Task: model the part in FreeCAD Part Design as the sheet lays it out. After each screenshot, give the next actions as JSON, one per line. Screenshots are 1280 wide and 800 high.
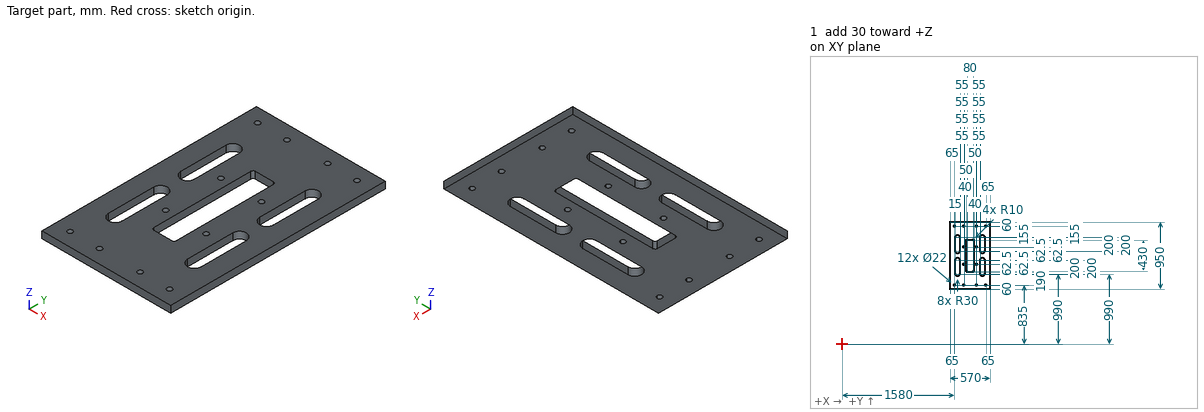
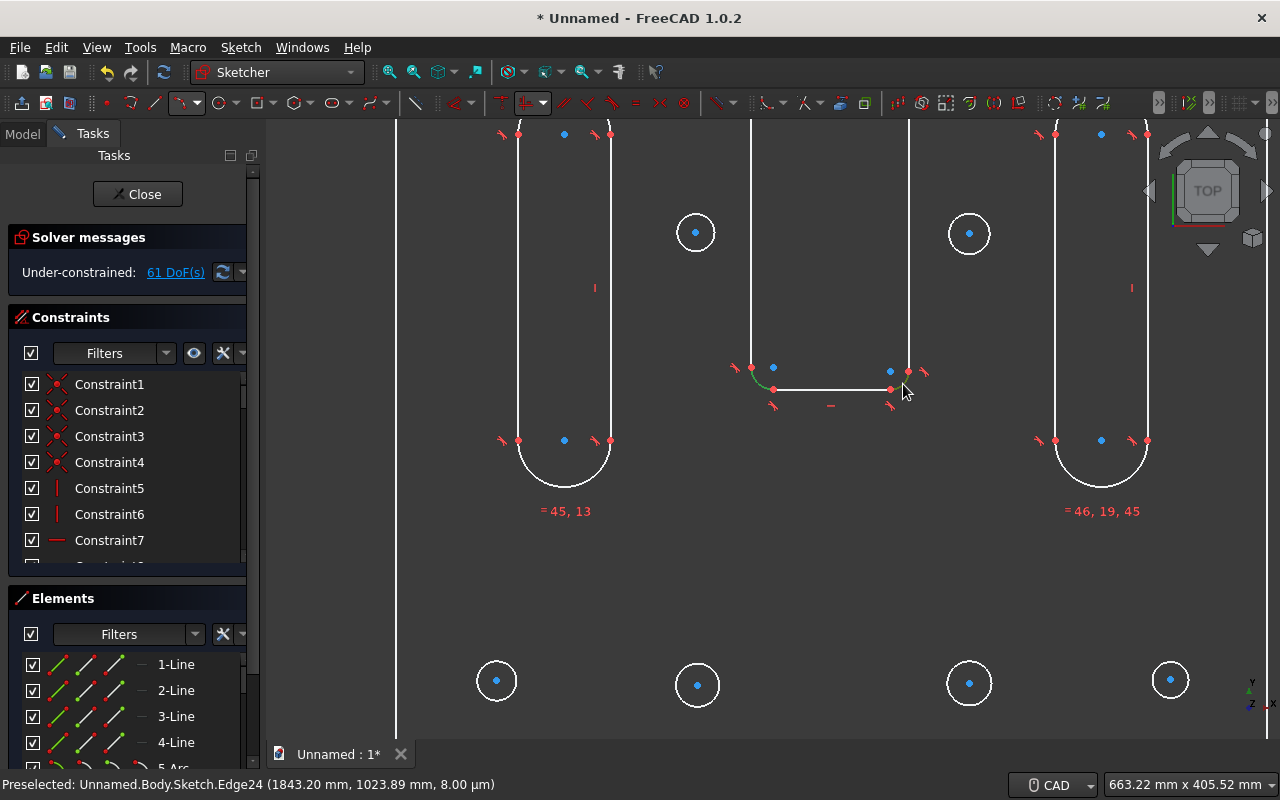
{"action": "left_click", "coordinate": [636, 104]}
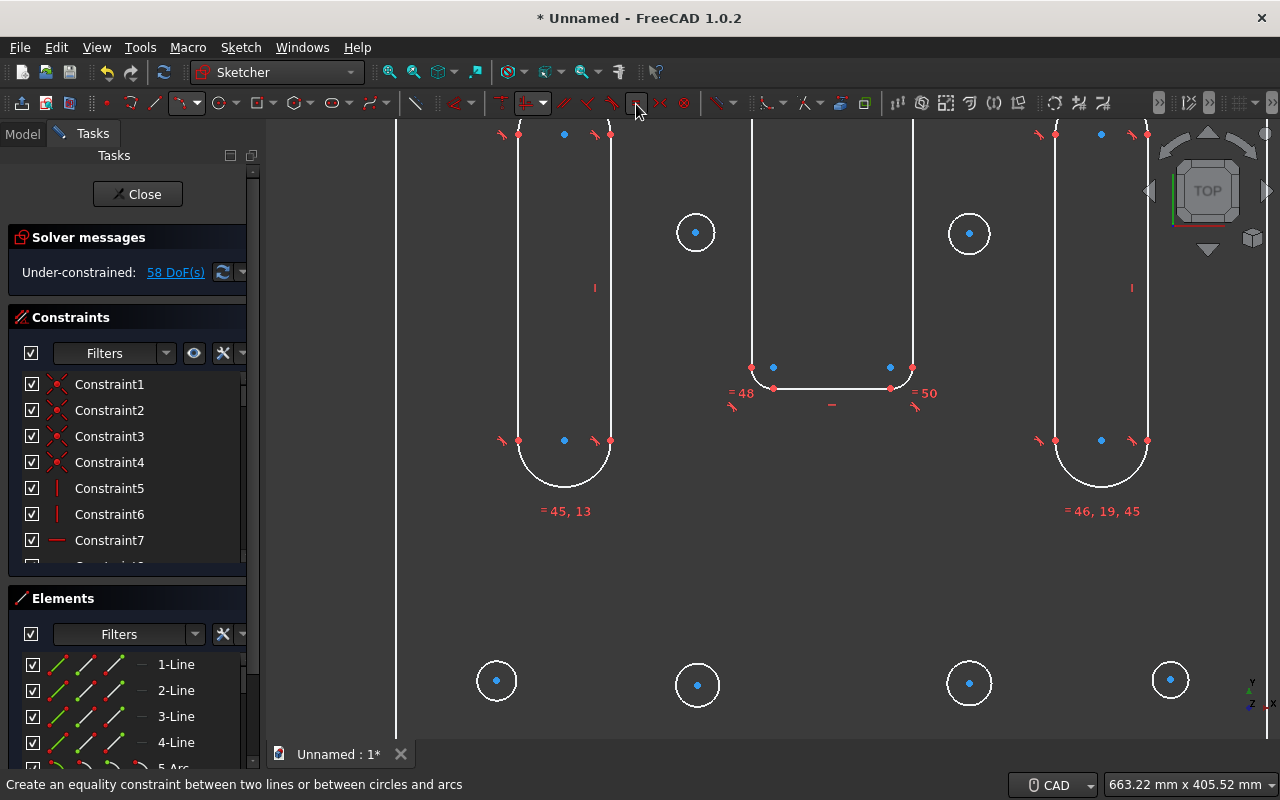
{"action": "left_click", "coordinate": [511, 667]}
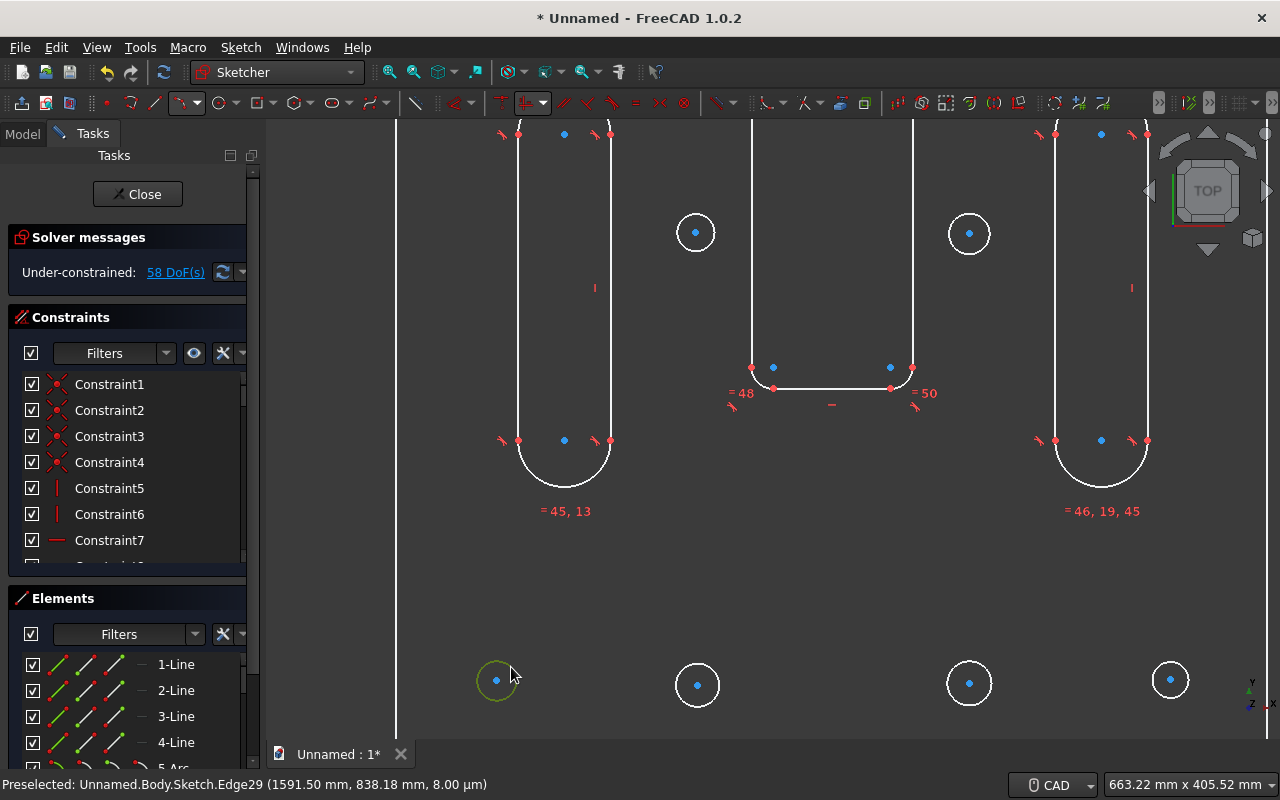
{"action": "left_click", "coordinate": [713, 670]}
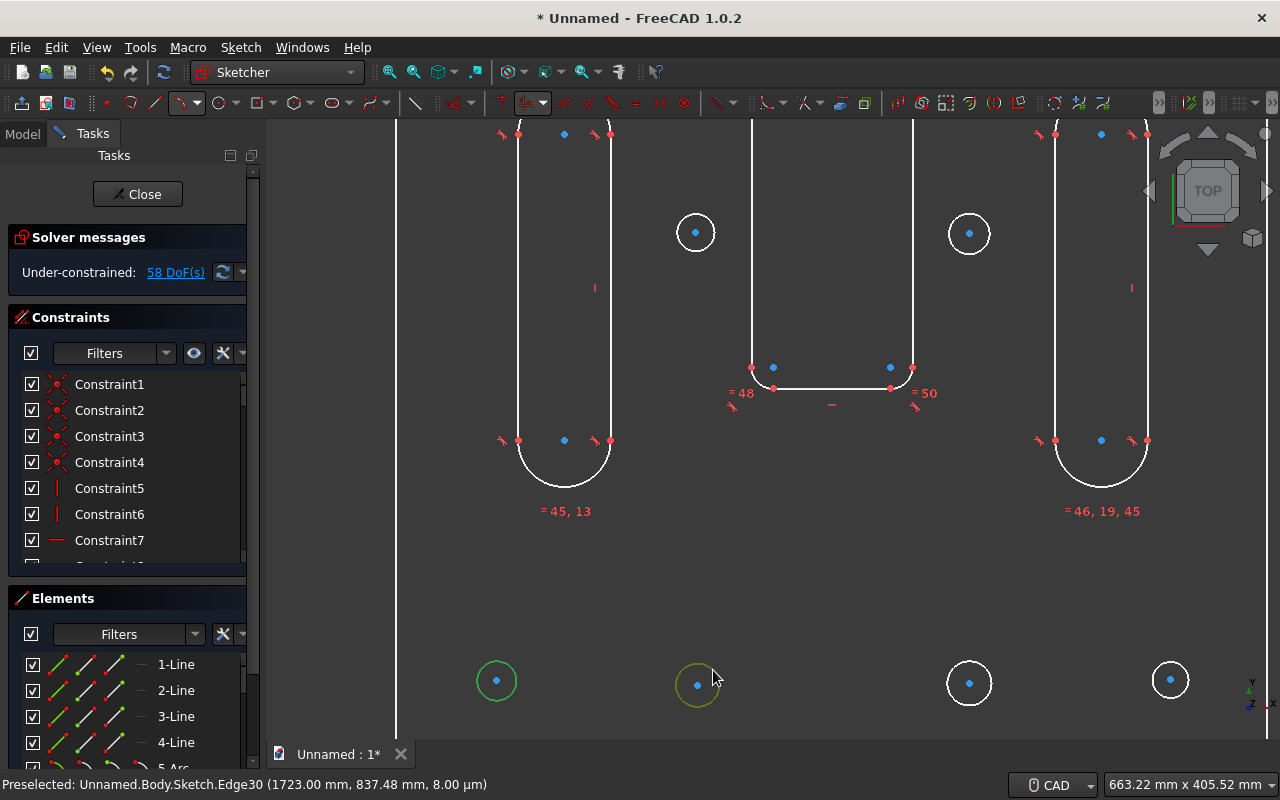
{"action": "left_click", "coordinate": [709, 219]}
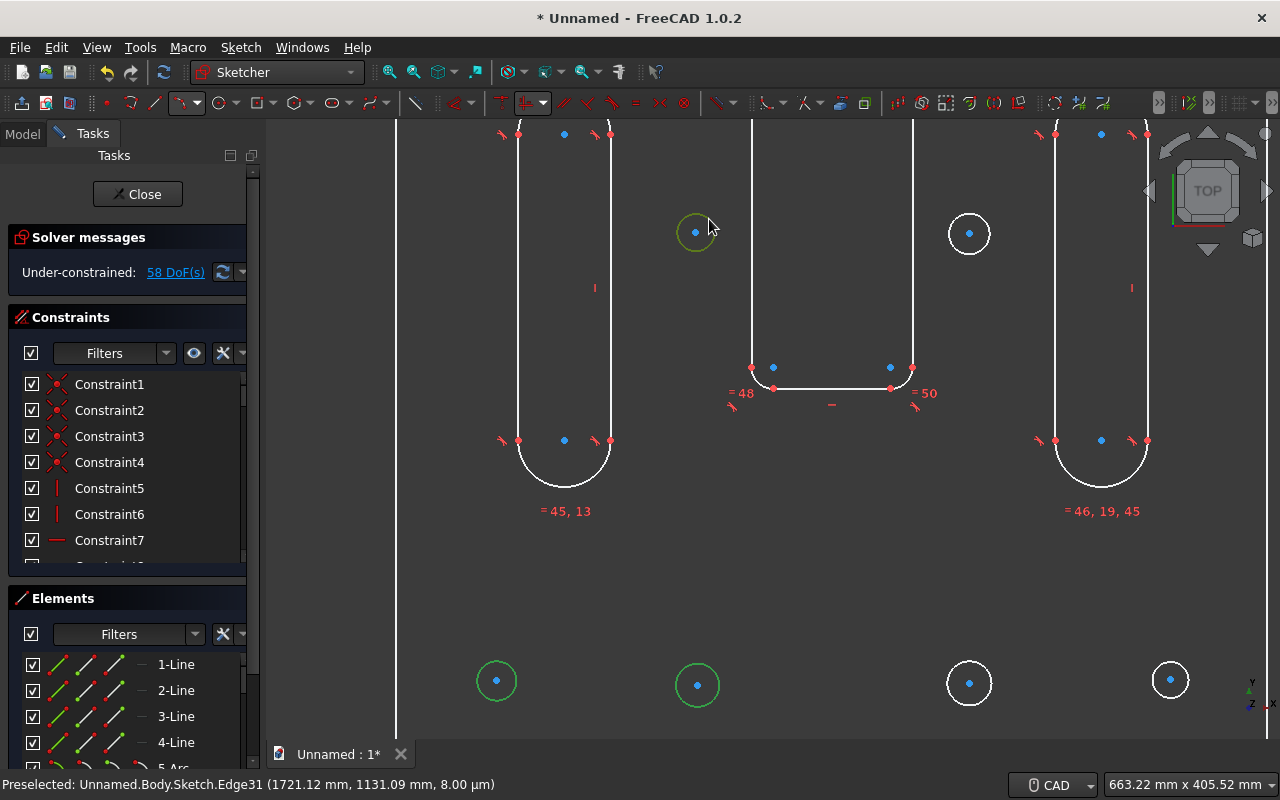
{"action": "left_click", "coordinate": [985, 668]}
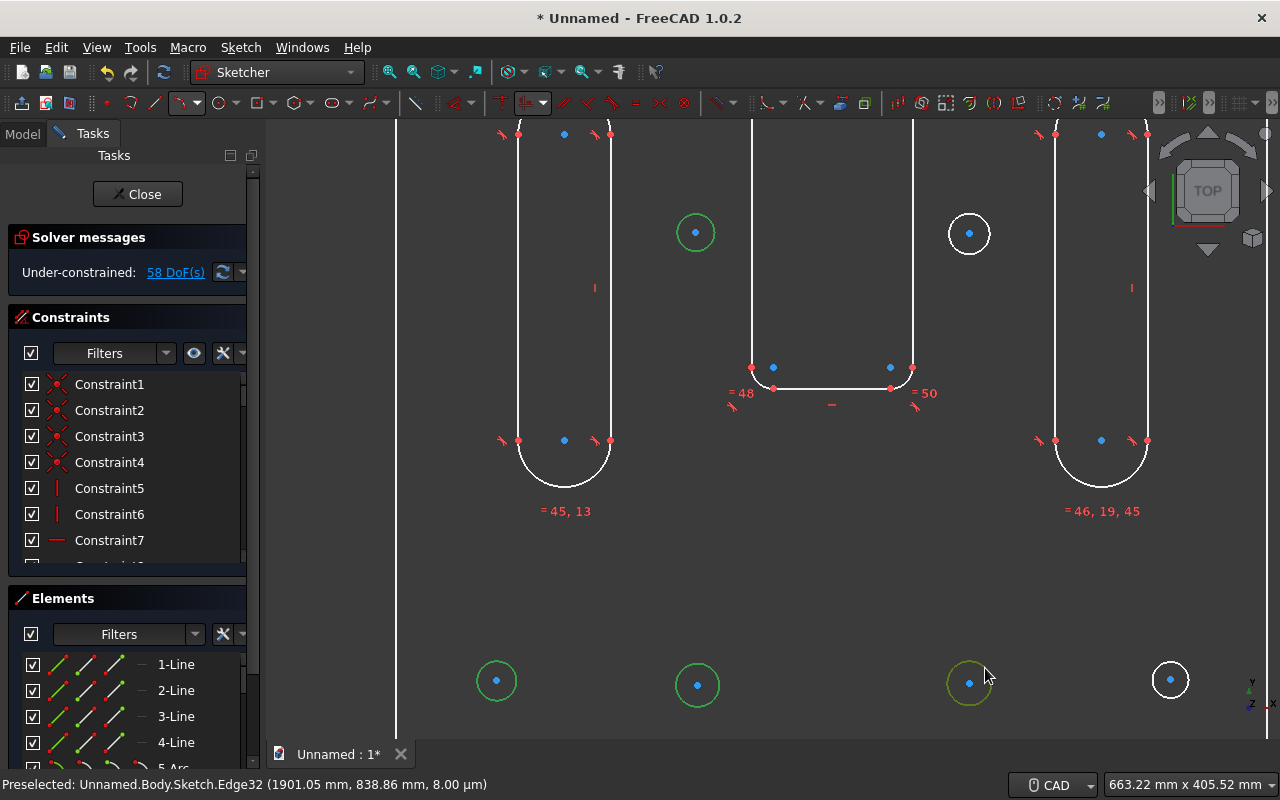
{"action": "scroll", "coordinate": [908, 388], "scroll_direction": "down", "scroll_amount": 9}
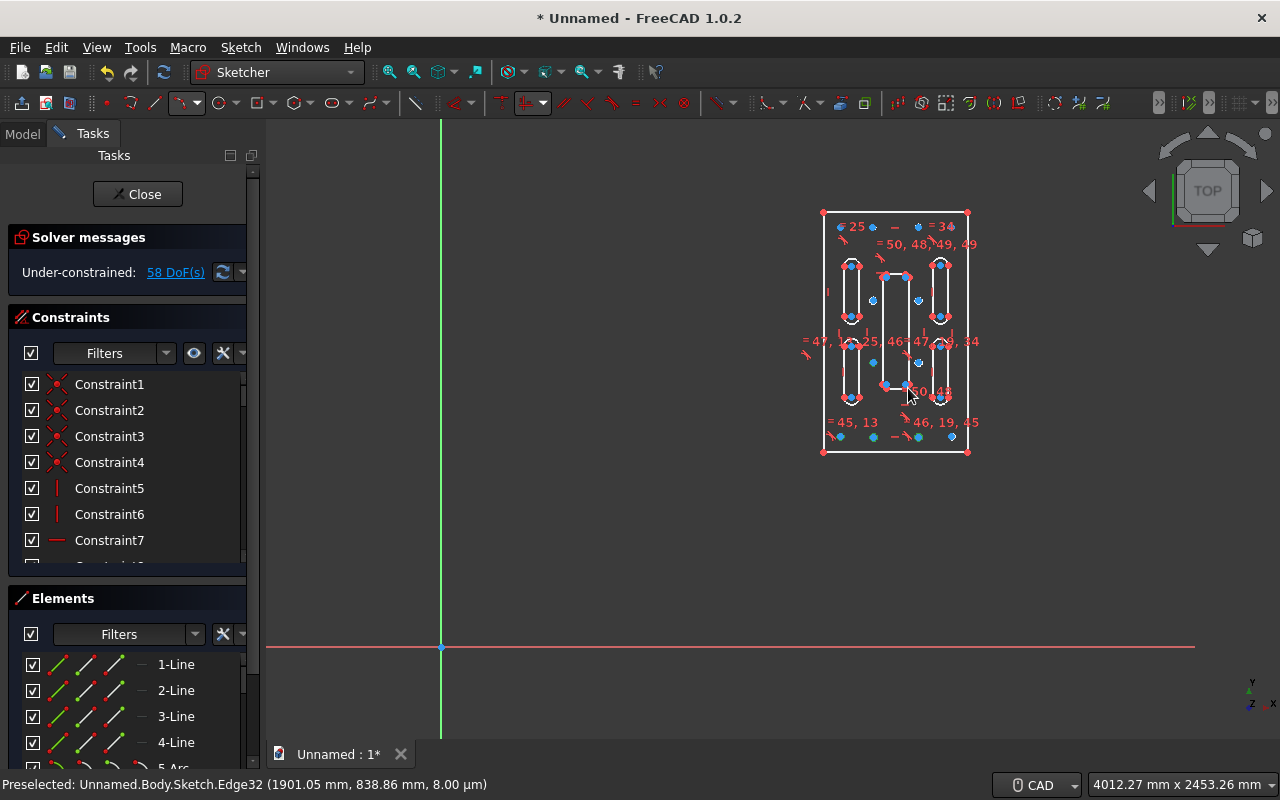
{"action": "scroll", "coordinate": [954, 435], "scroll_direction": "up", "scroll_amount": 8}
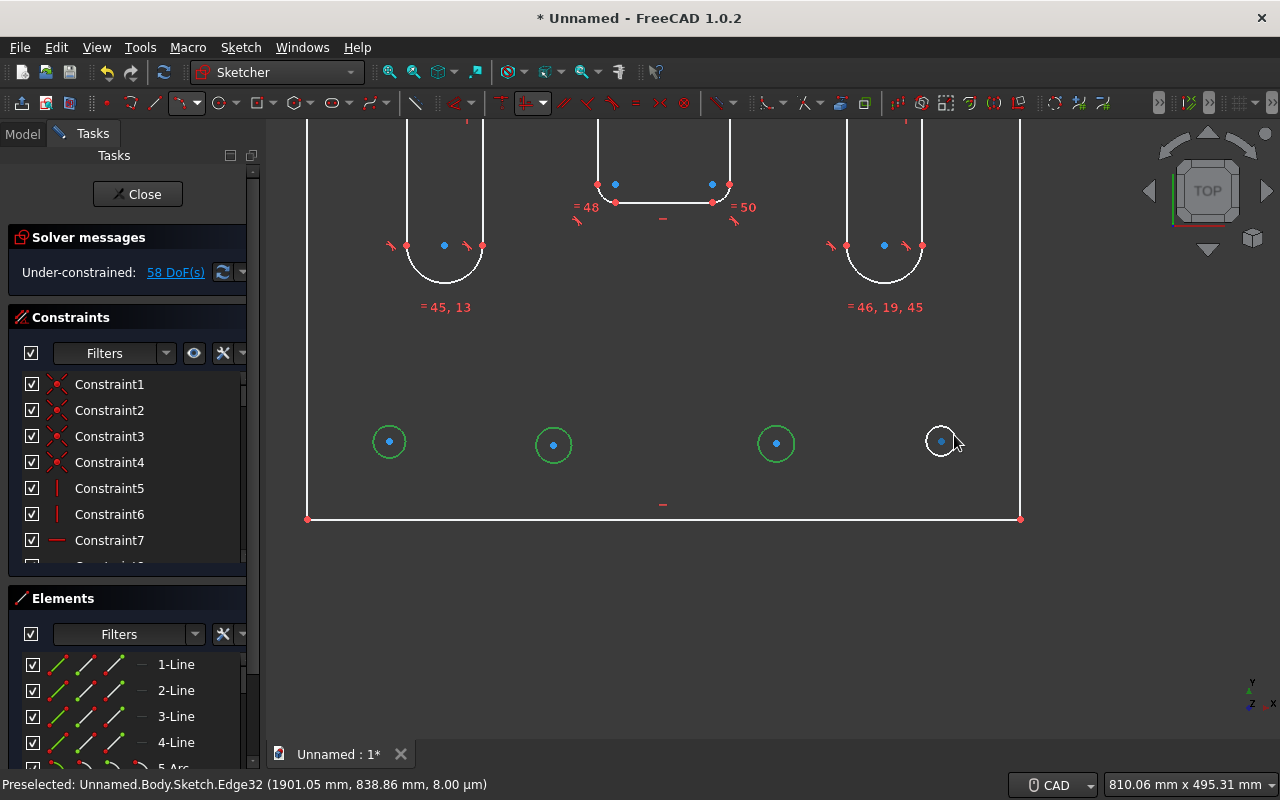
{"action": "left_click", "coordinate": [951, 431]}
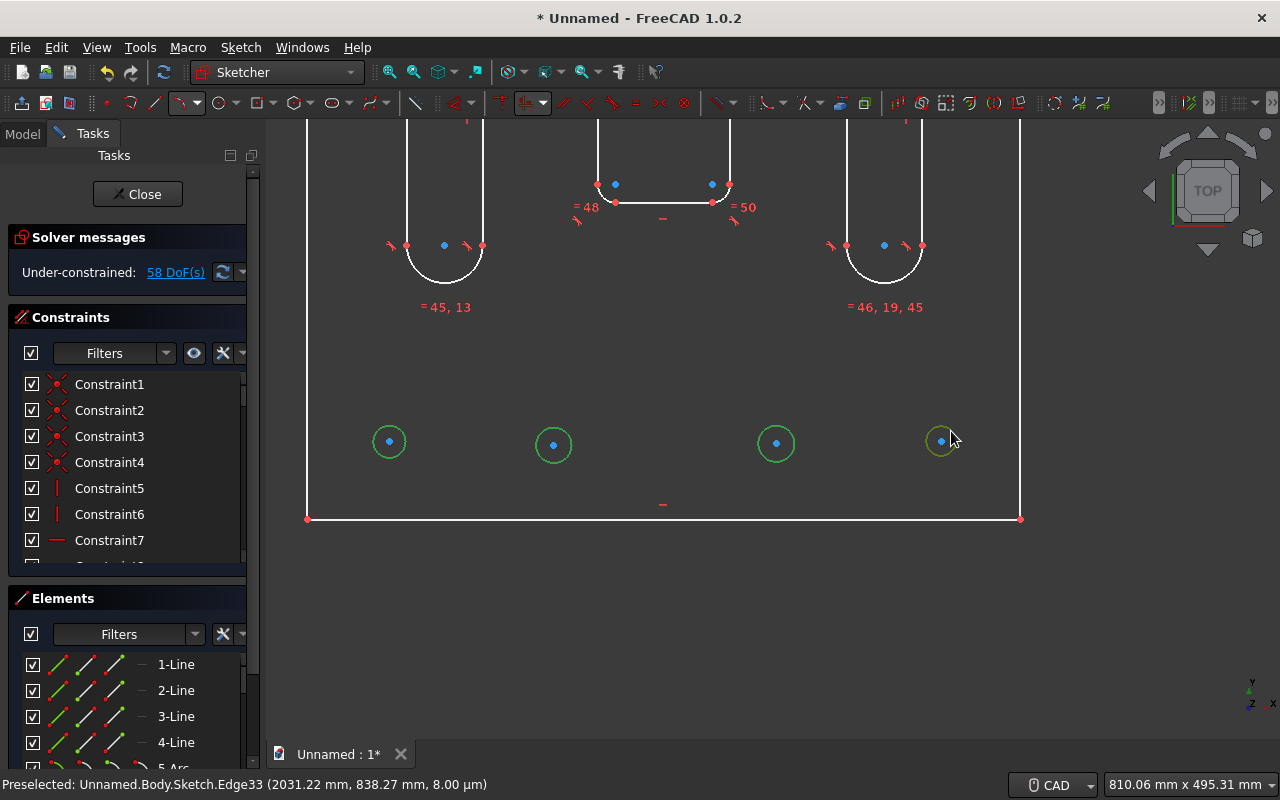
{"action": "scroll", "coordinate": [954, 435], "scroll_direction": "down", "scroll_amount": 8}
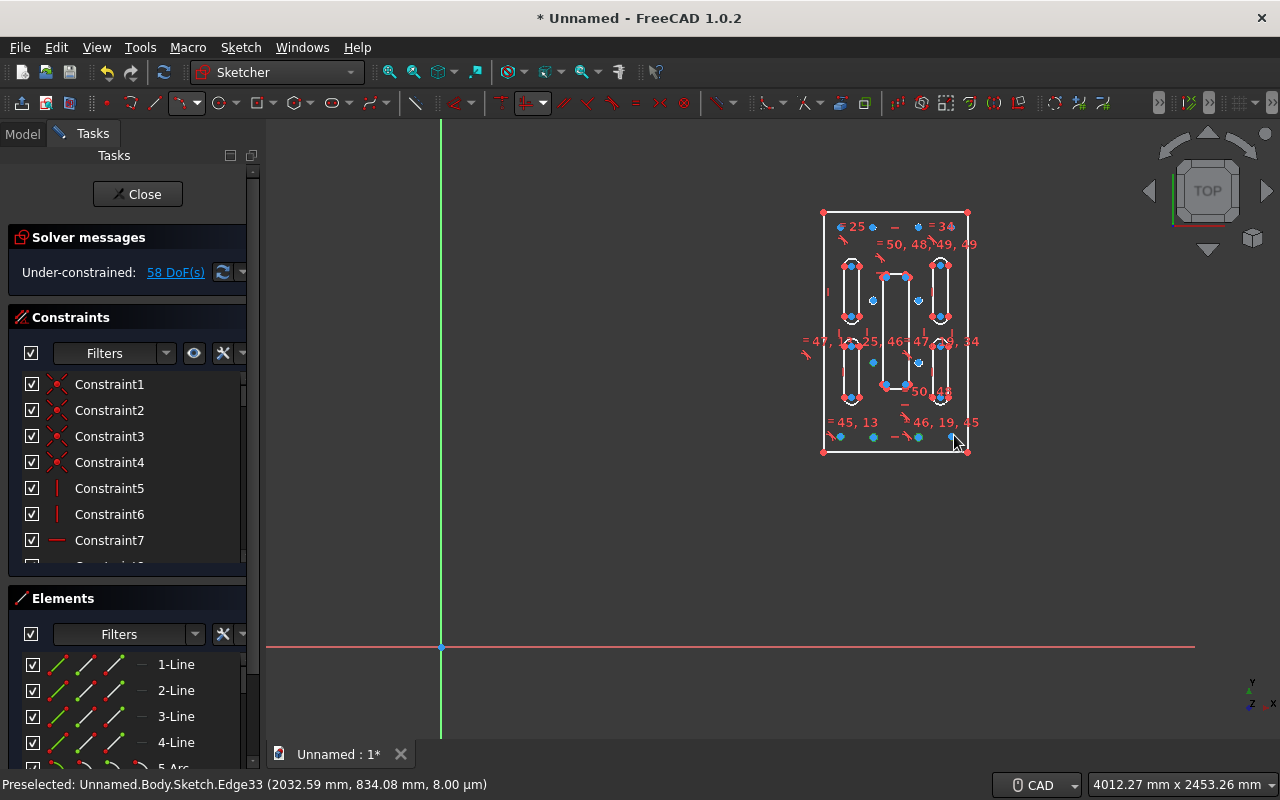
{"action": "scroll", "coordinate": [921, 361], "scroll_direction": "up", "scroll_amount": 8}